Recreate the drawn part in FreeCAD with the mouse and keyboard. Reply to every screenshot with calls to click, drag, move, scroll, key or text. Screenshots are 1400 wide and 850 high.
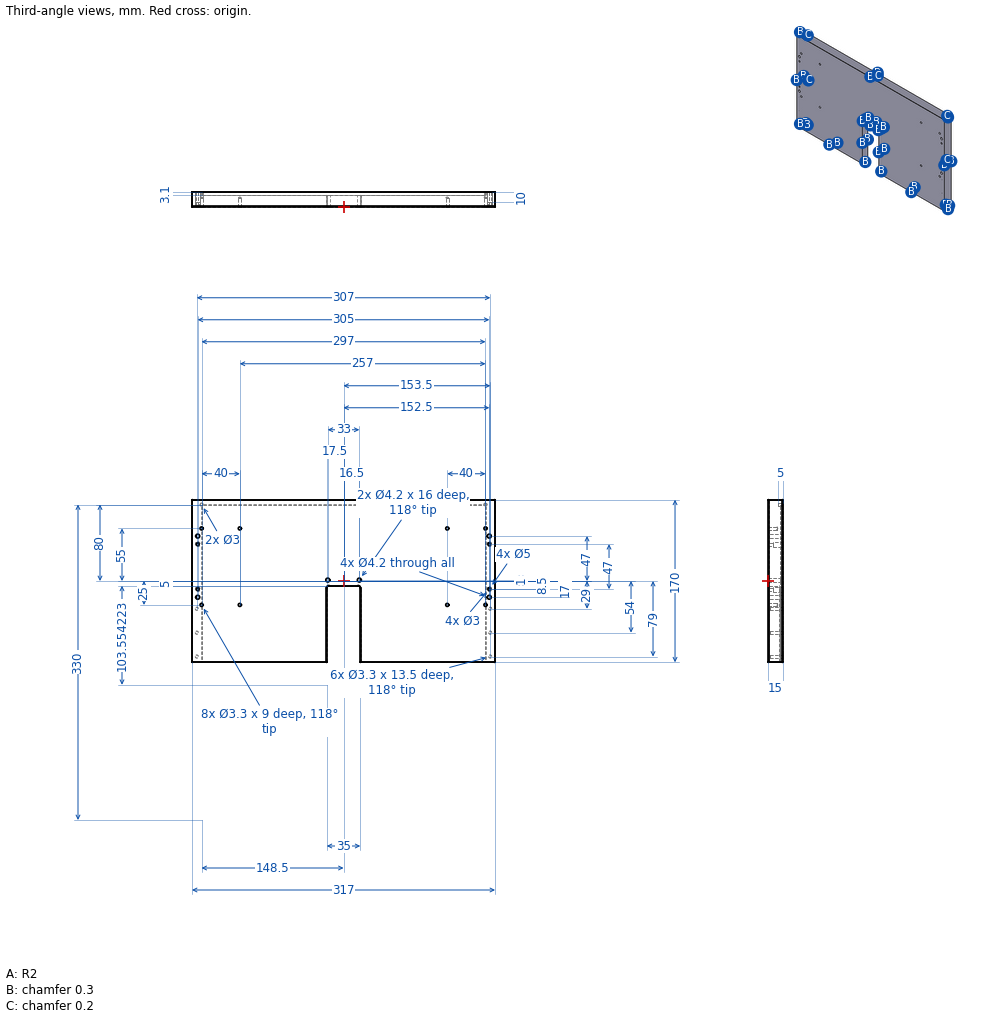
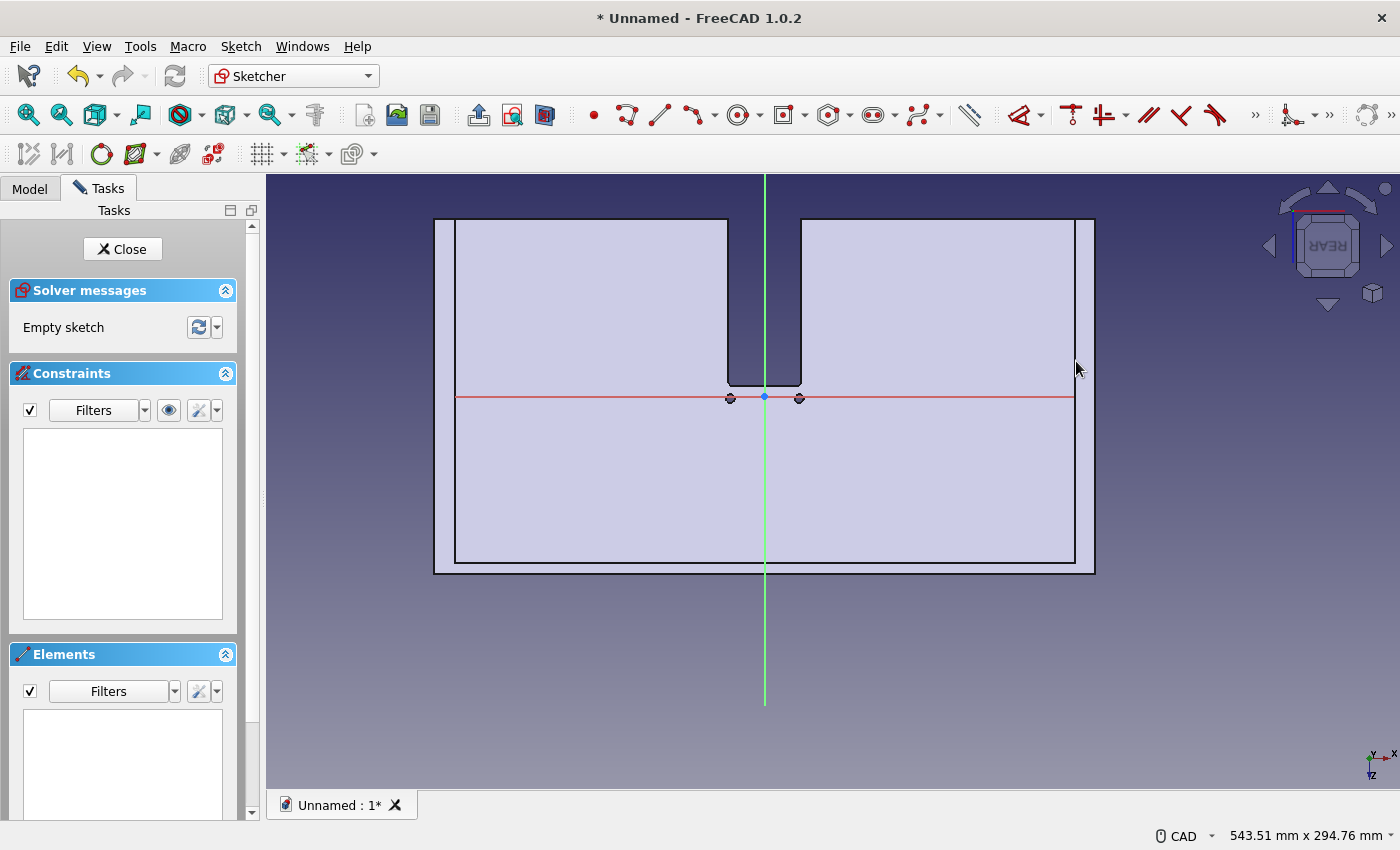
key(g)
key(c)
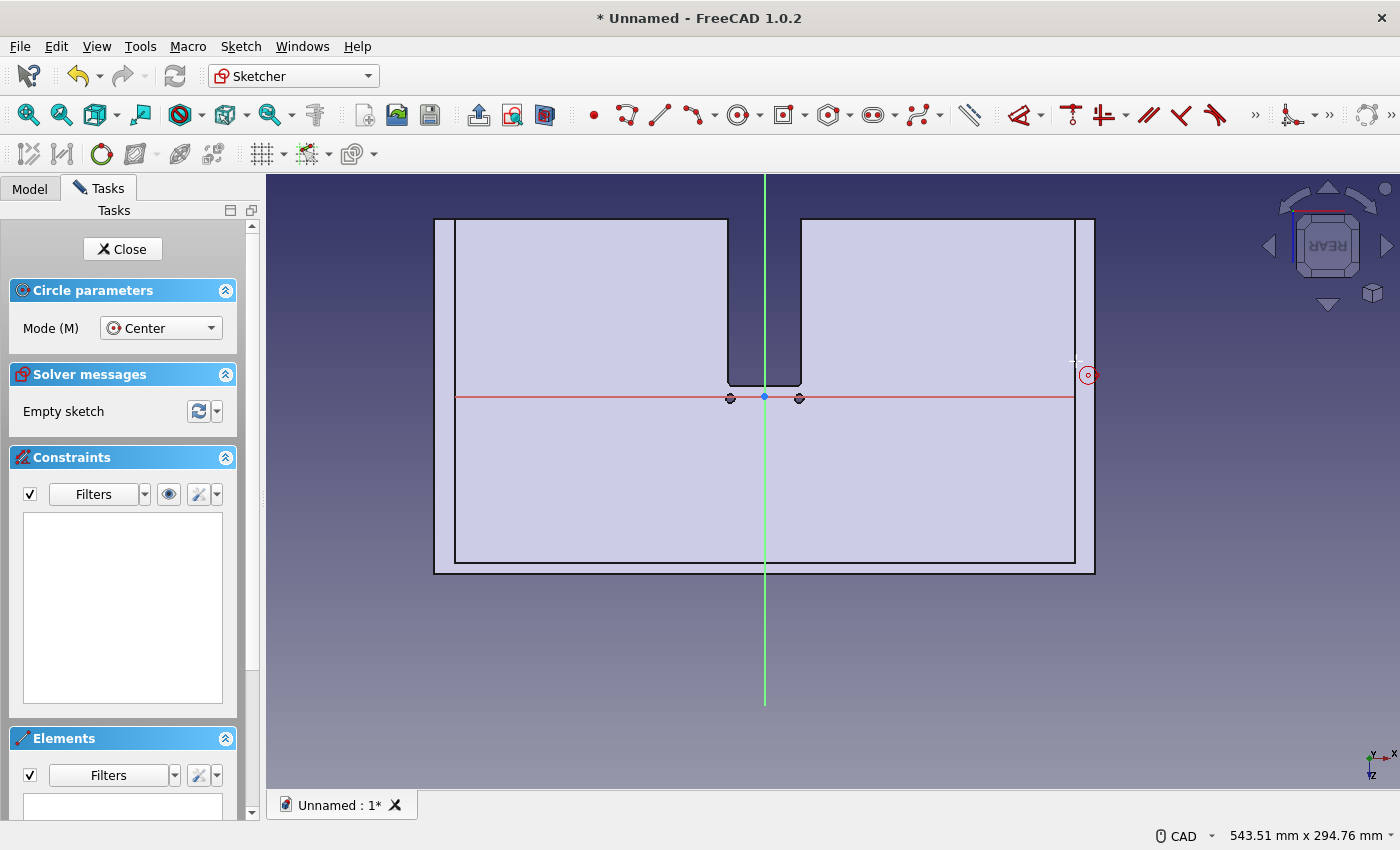
scroll(455, 563, up, 10)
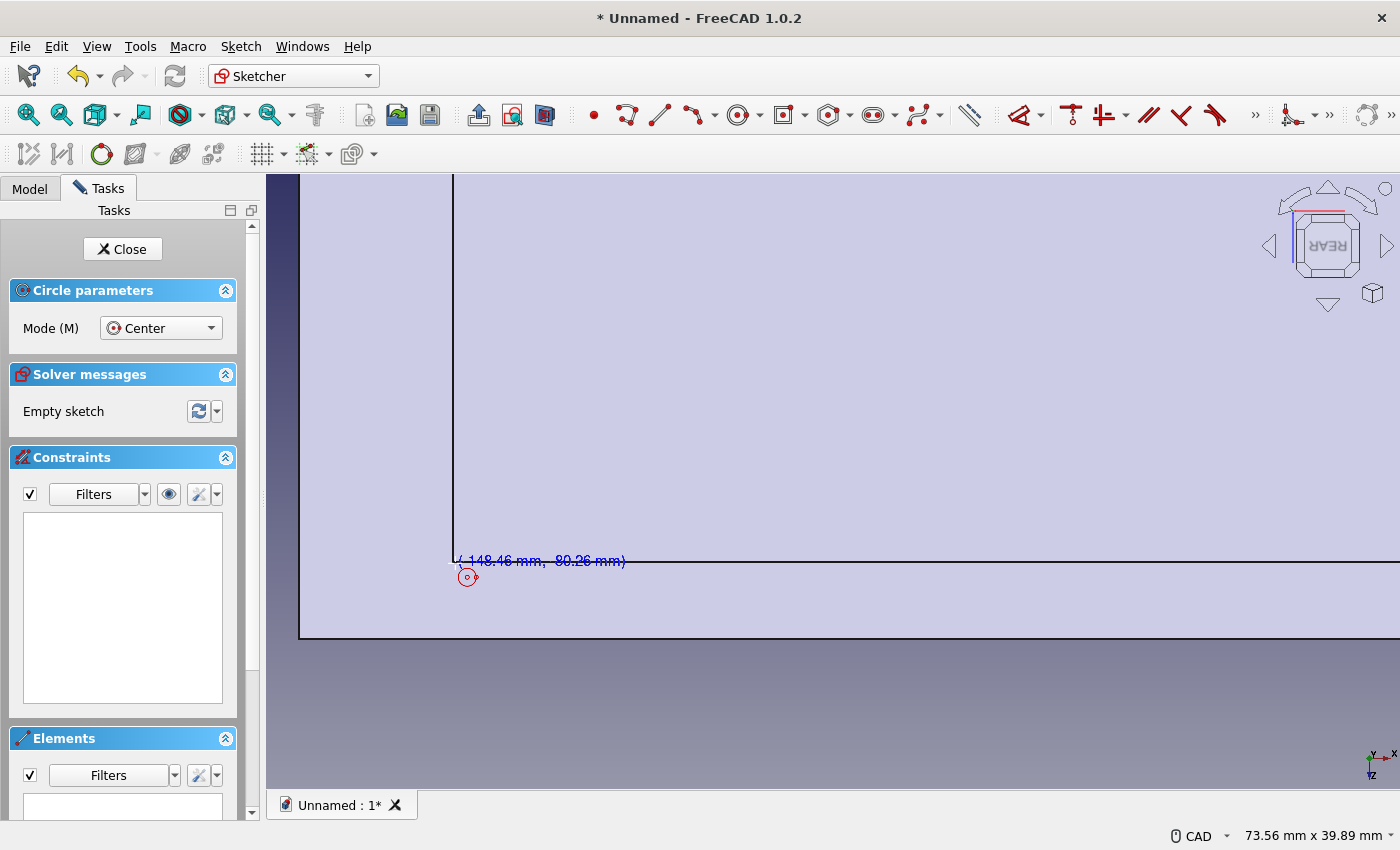
scroll(455, 564, down, 10)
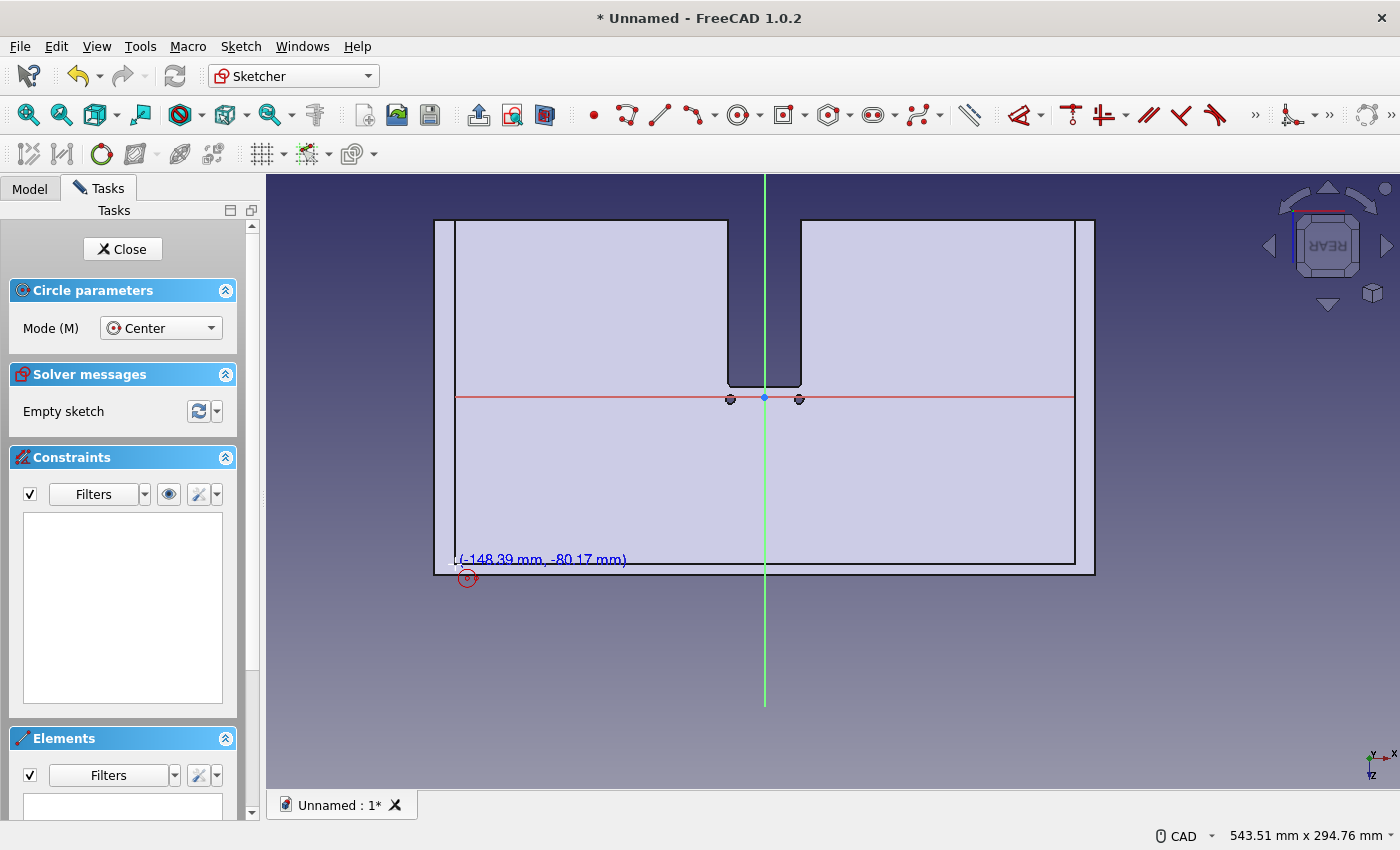
click(455, 564)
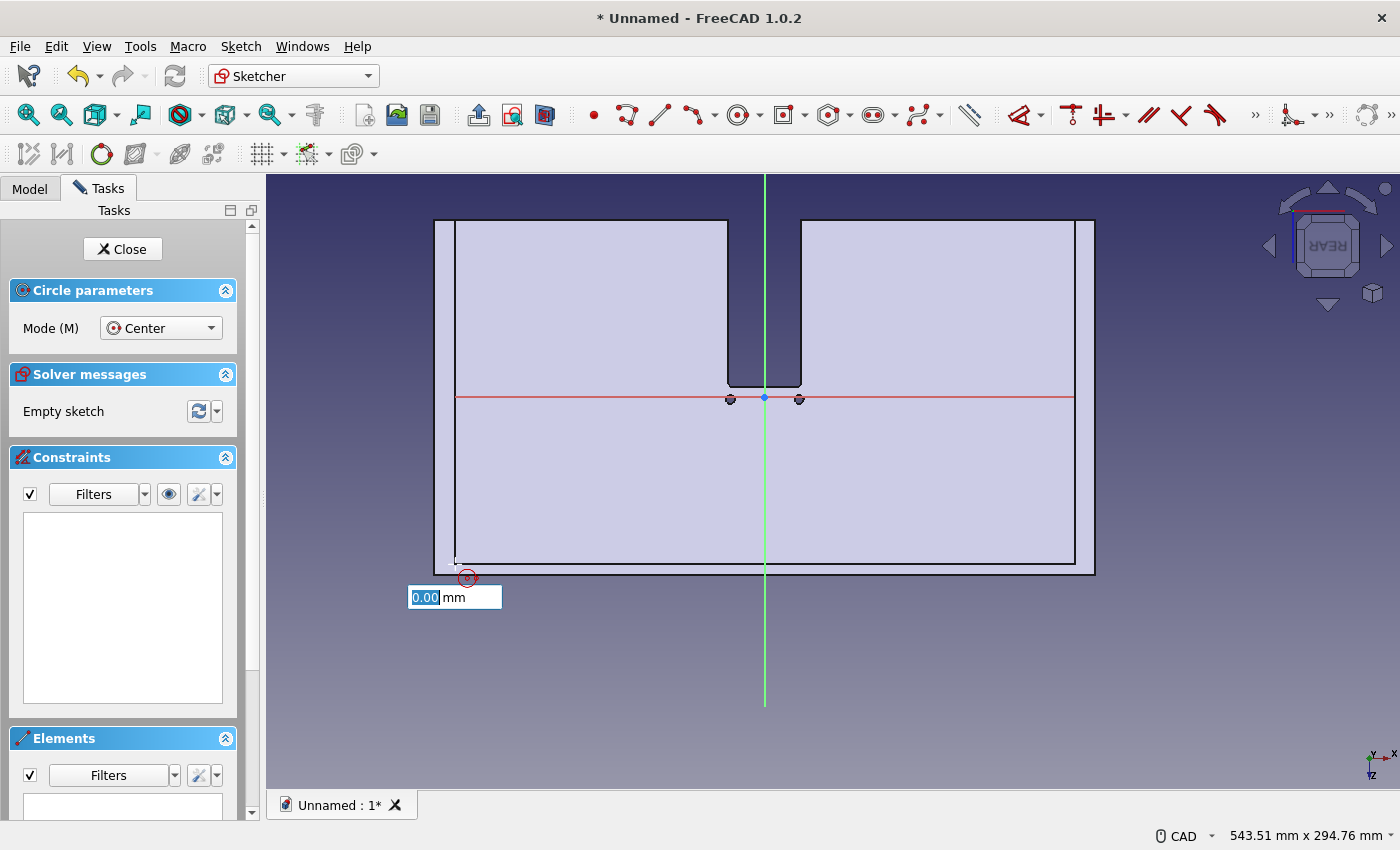
scroll(457, 562, up, 9)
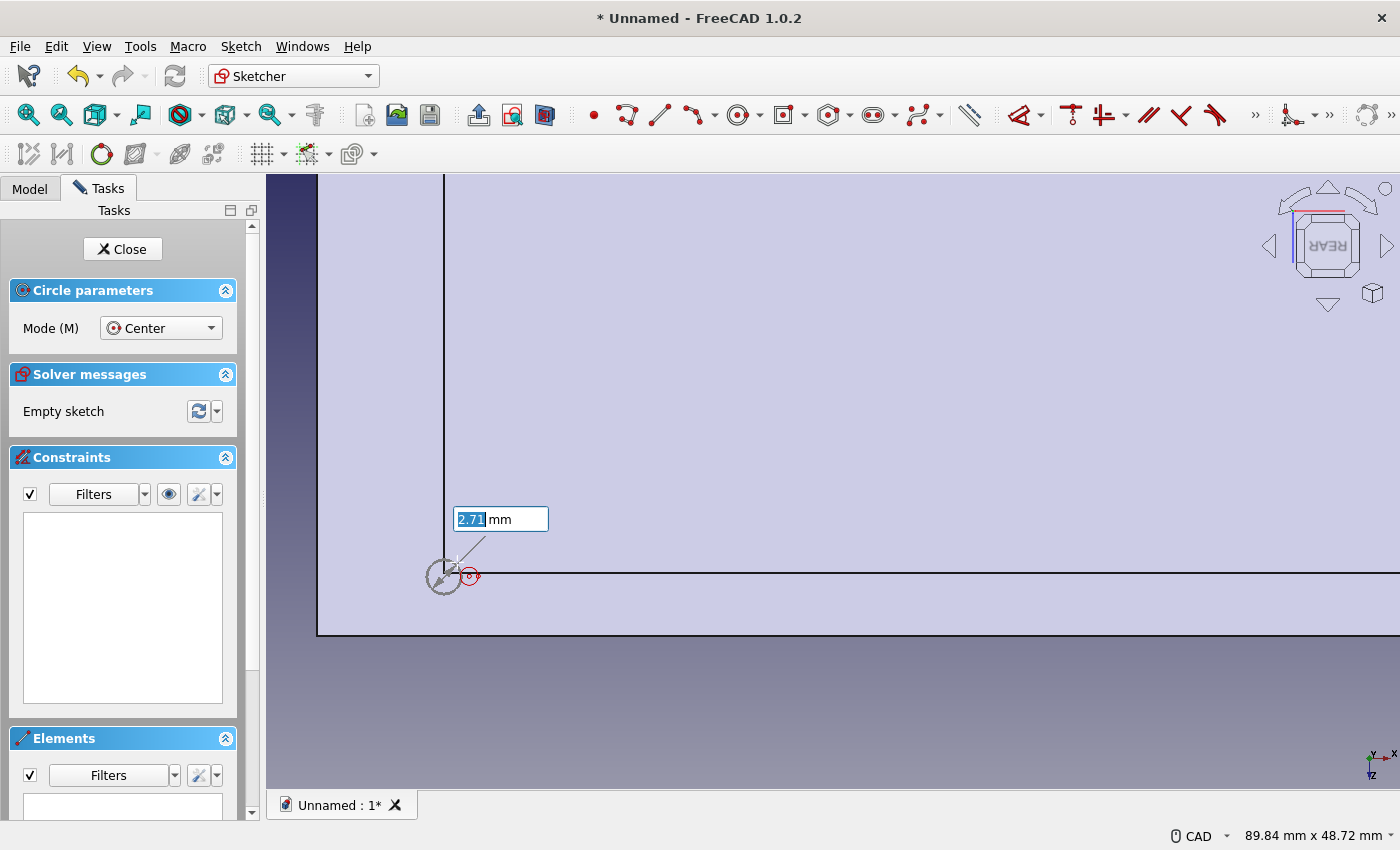
click(457, 560)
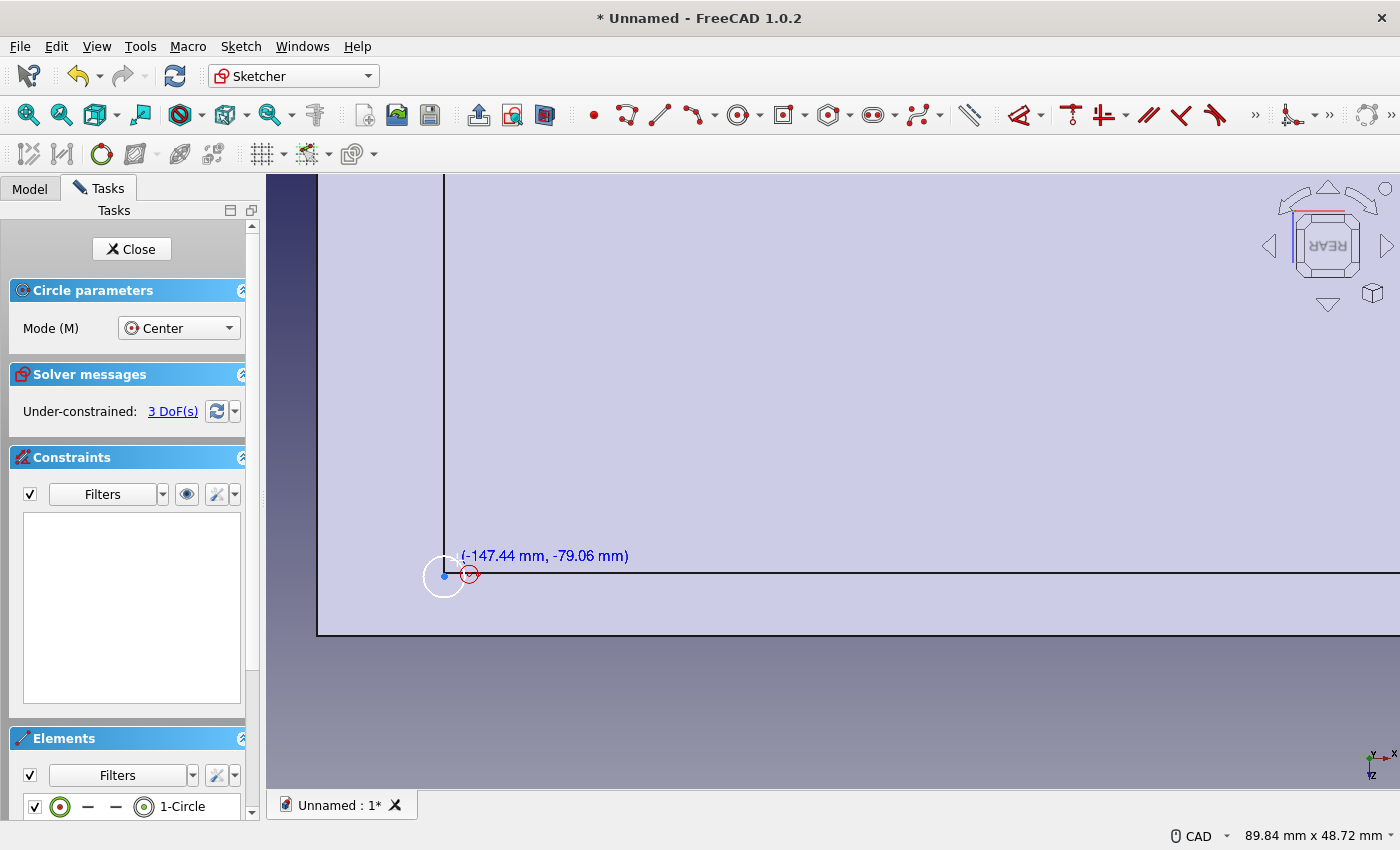
scroll(457, 562, down, 9)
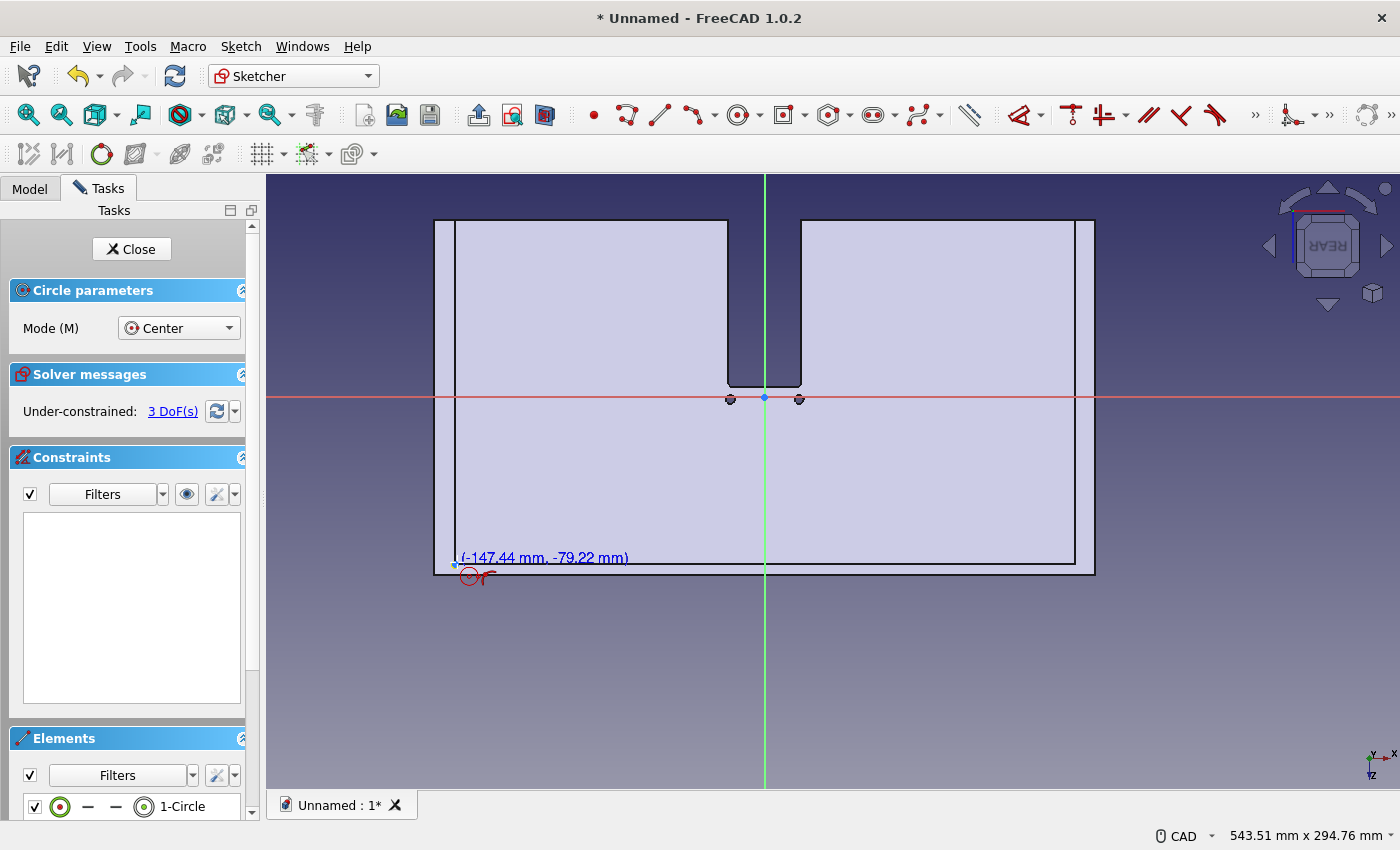
scroll(1075, 564, up, 10)